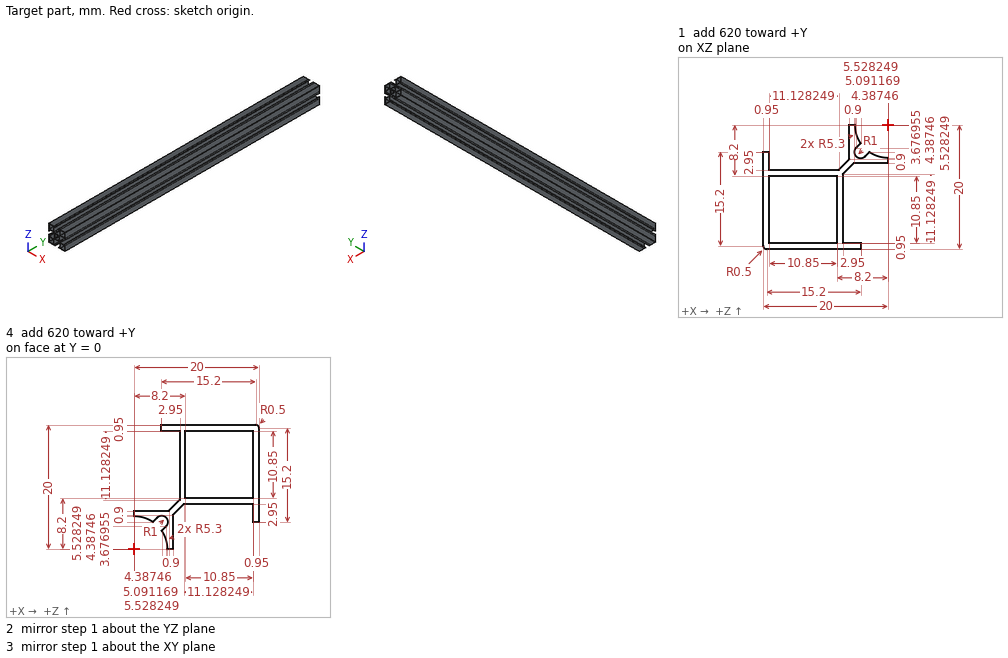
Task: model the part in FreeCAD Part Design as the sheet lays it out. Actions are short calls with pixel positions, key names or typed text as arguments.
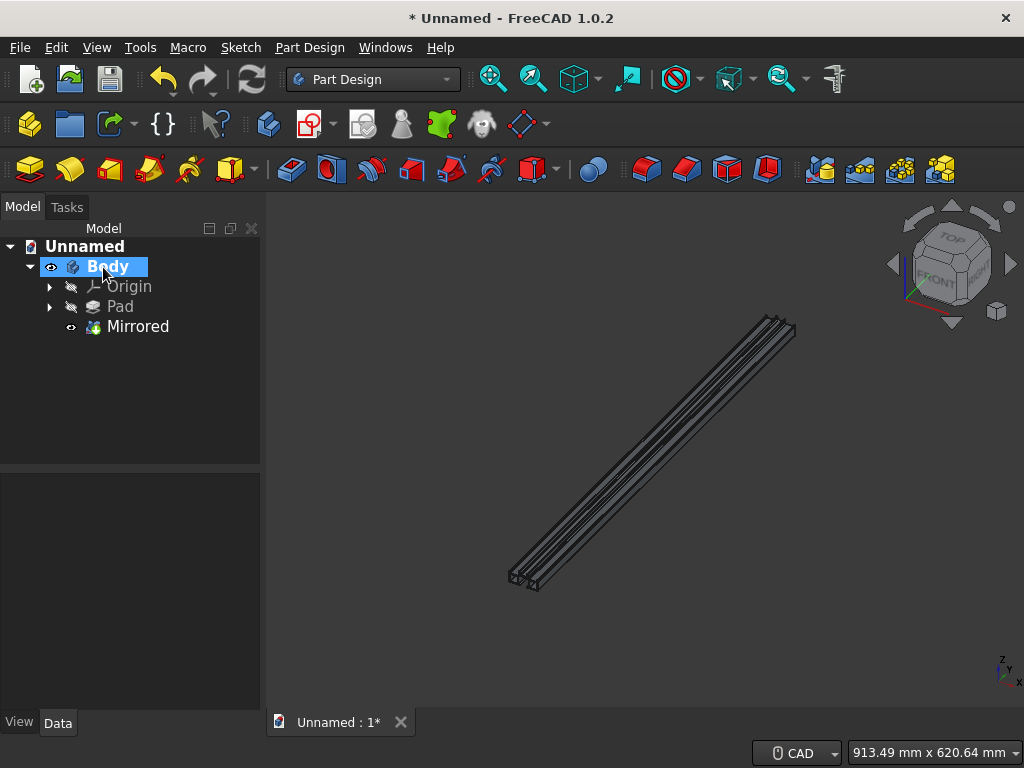
click(116, 307)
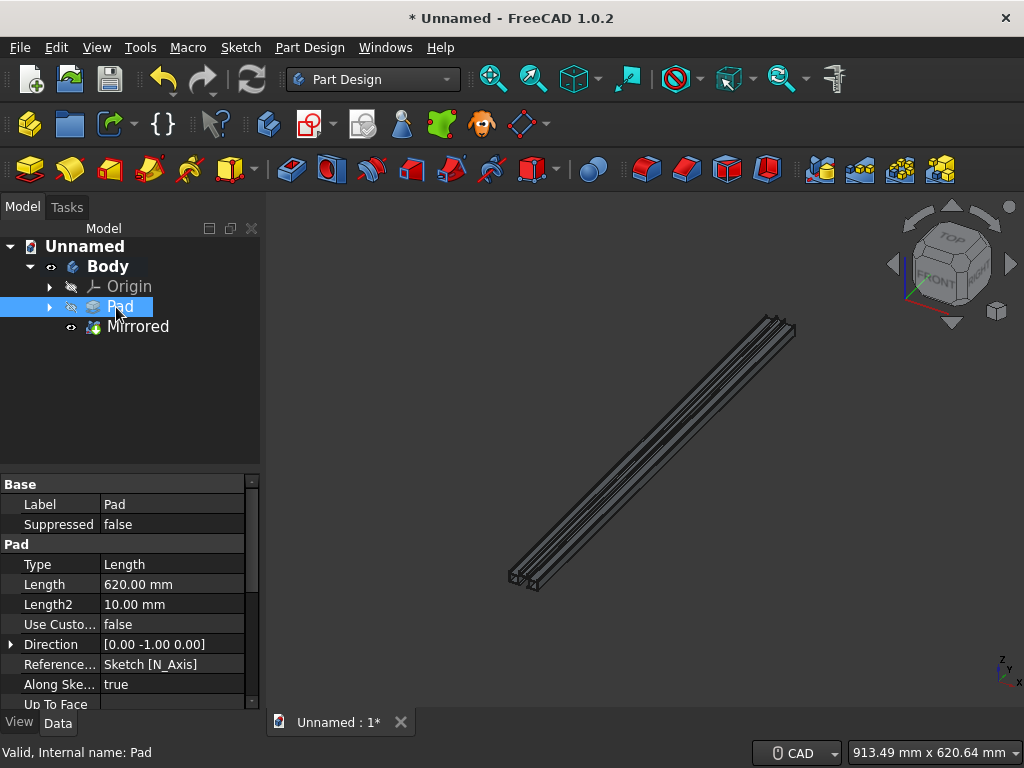
click(820, 170)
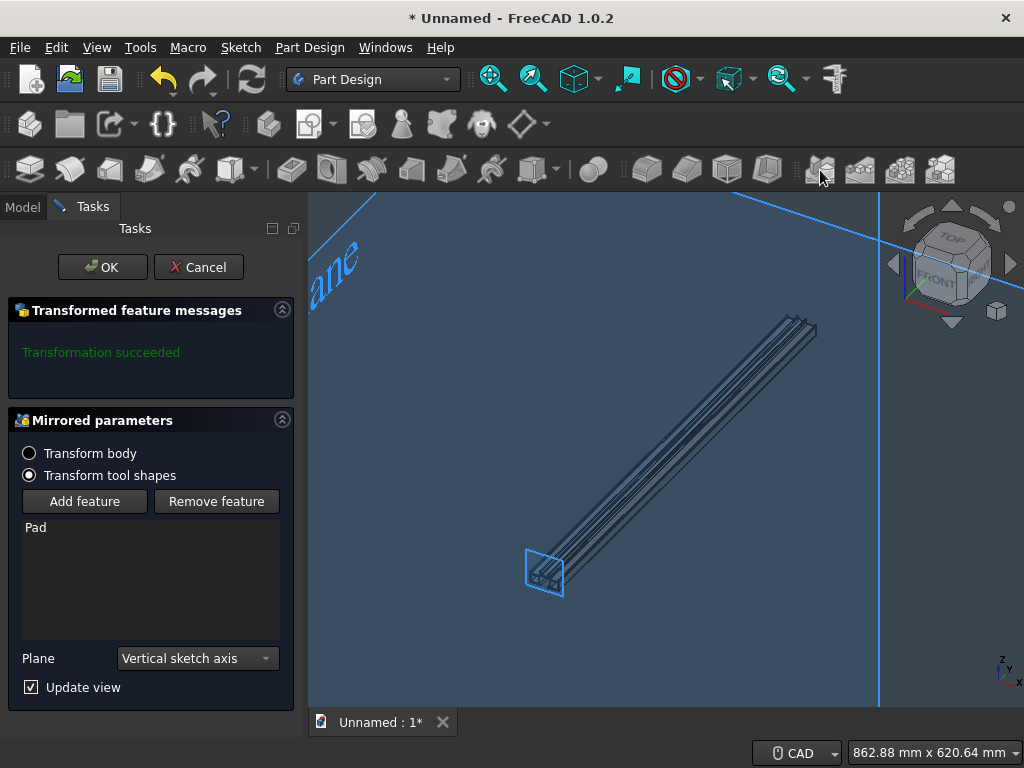
click(198, 658)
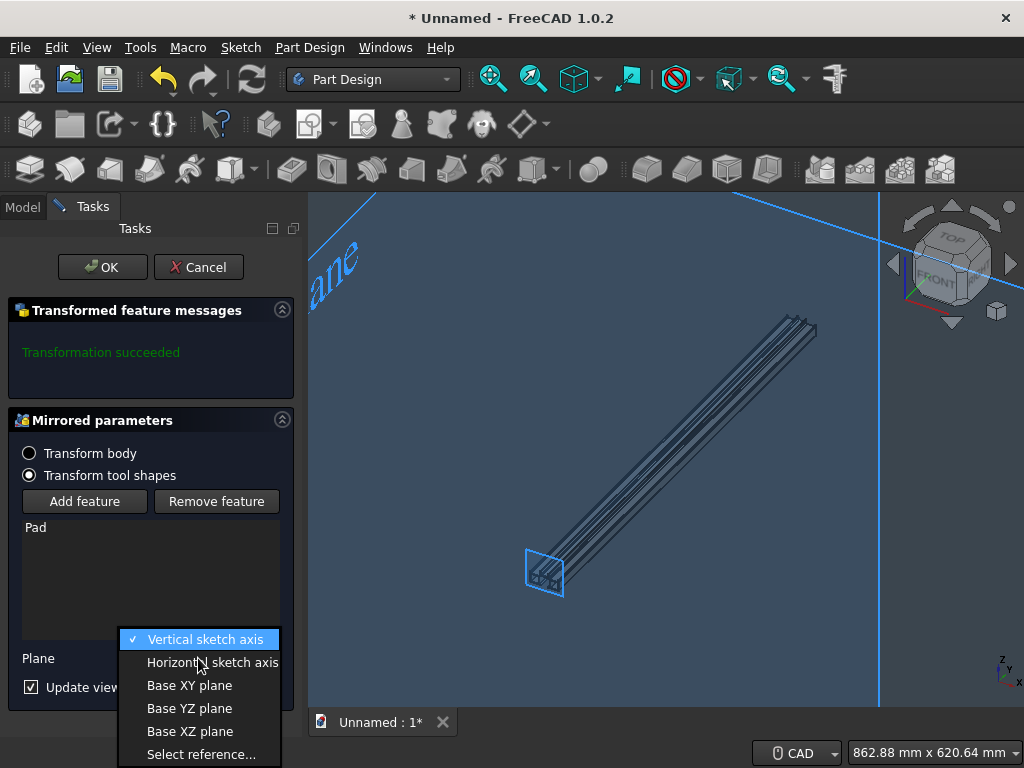
click(198, 686)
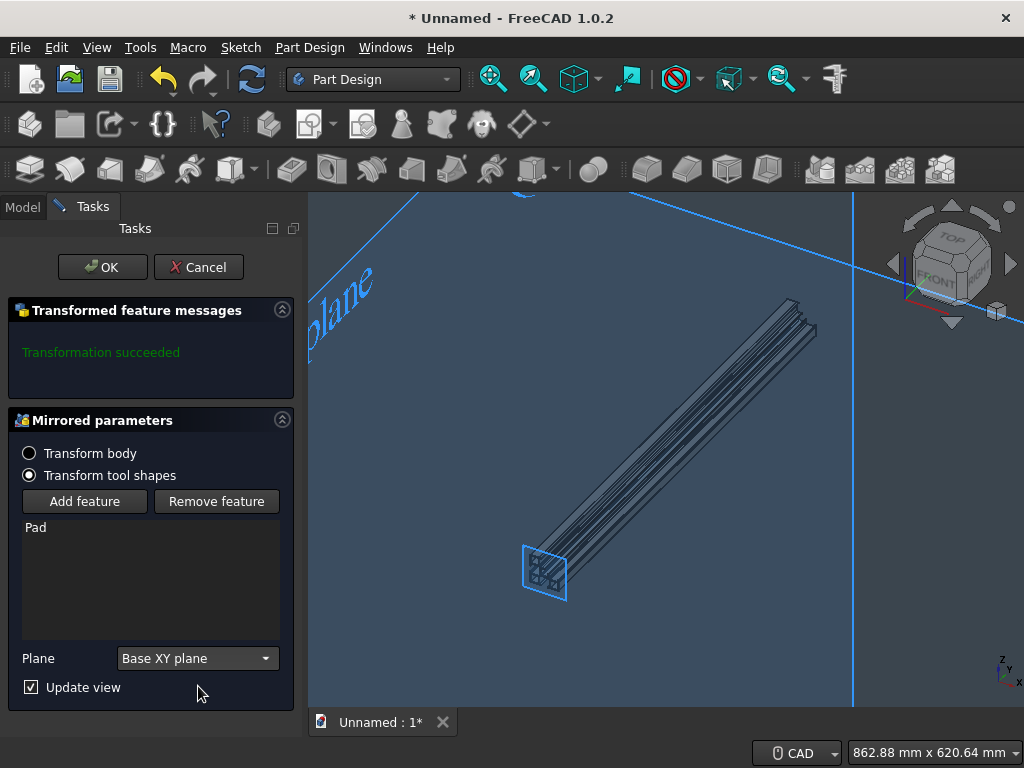
click(103, 267)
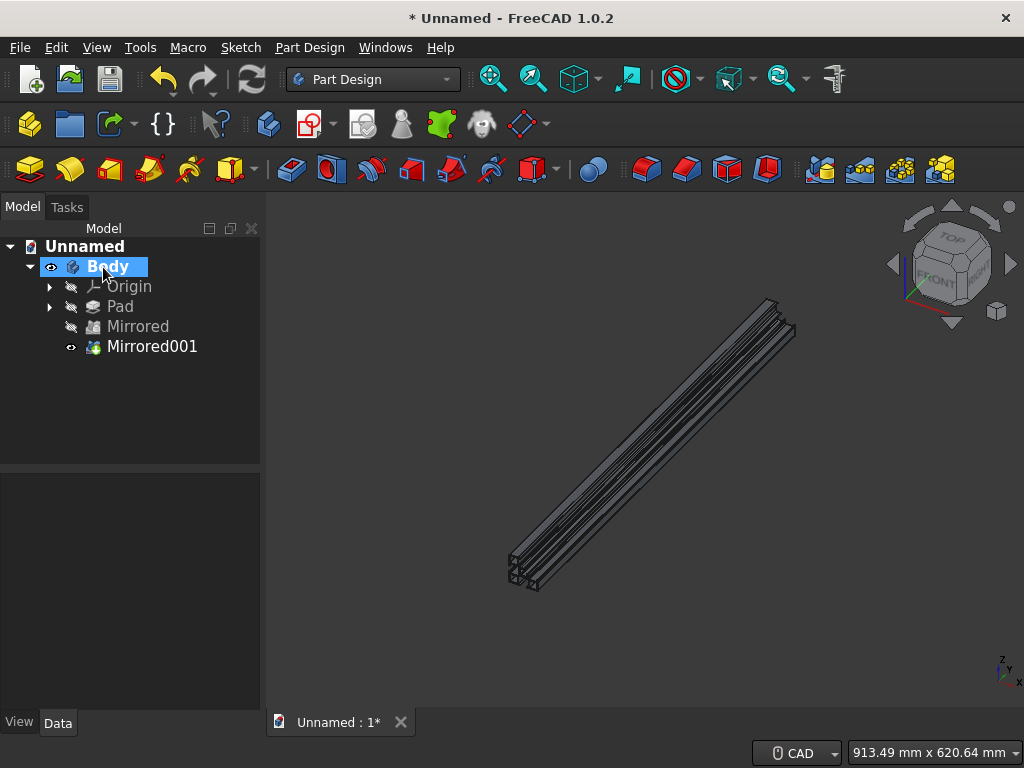
scroll(519, 574, up, 15)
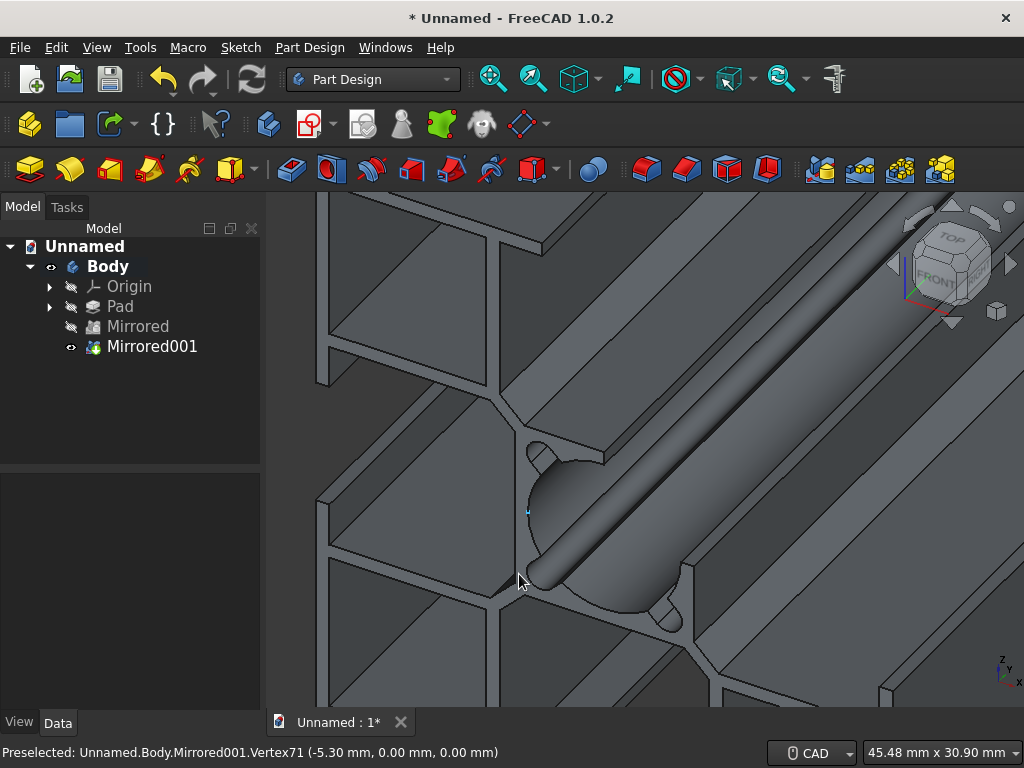
click(522, 587)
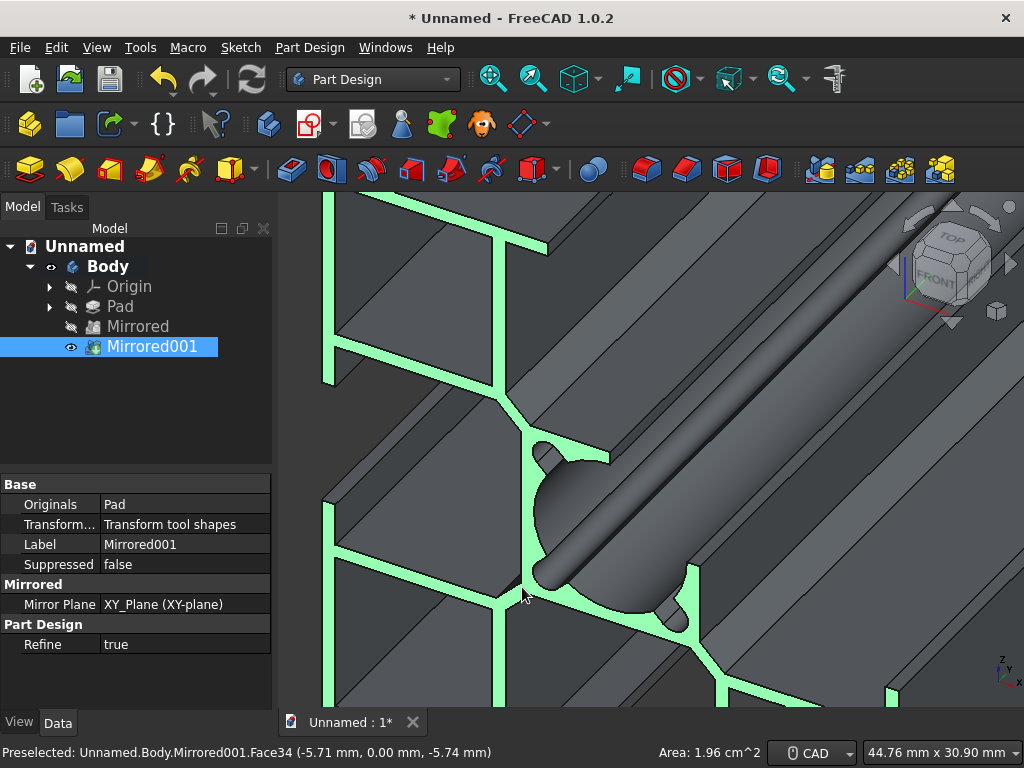
click(310, 124)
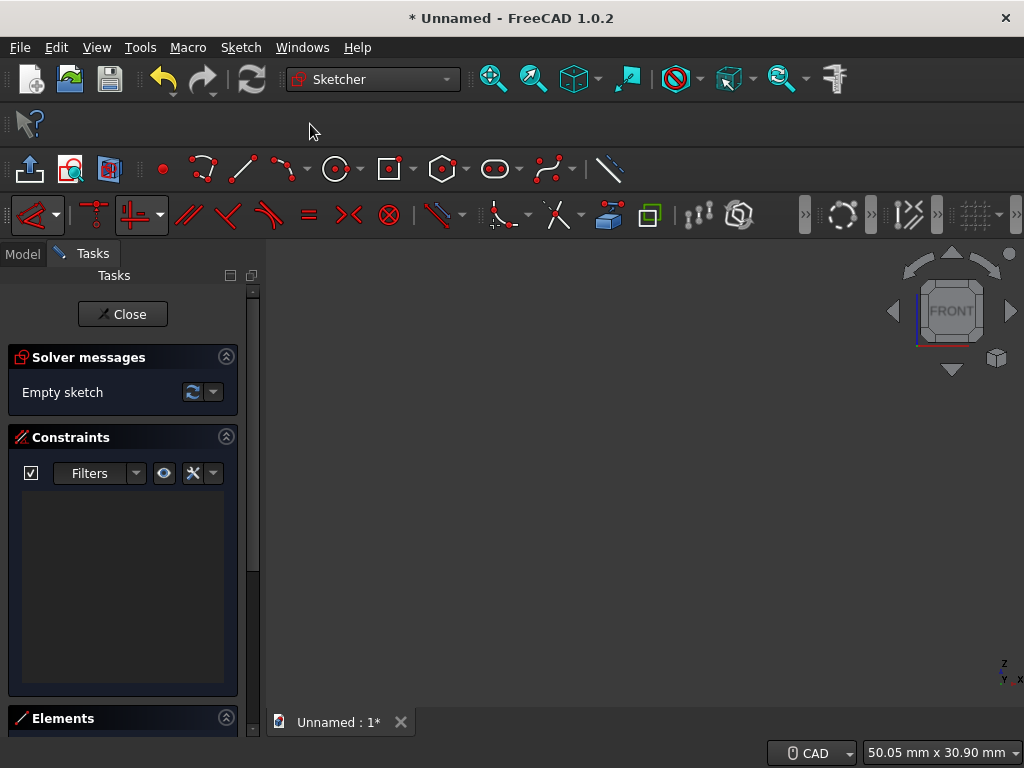
scroll(576, 473, down, 5)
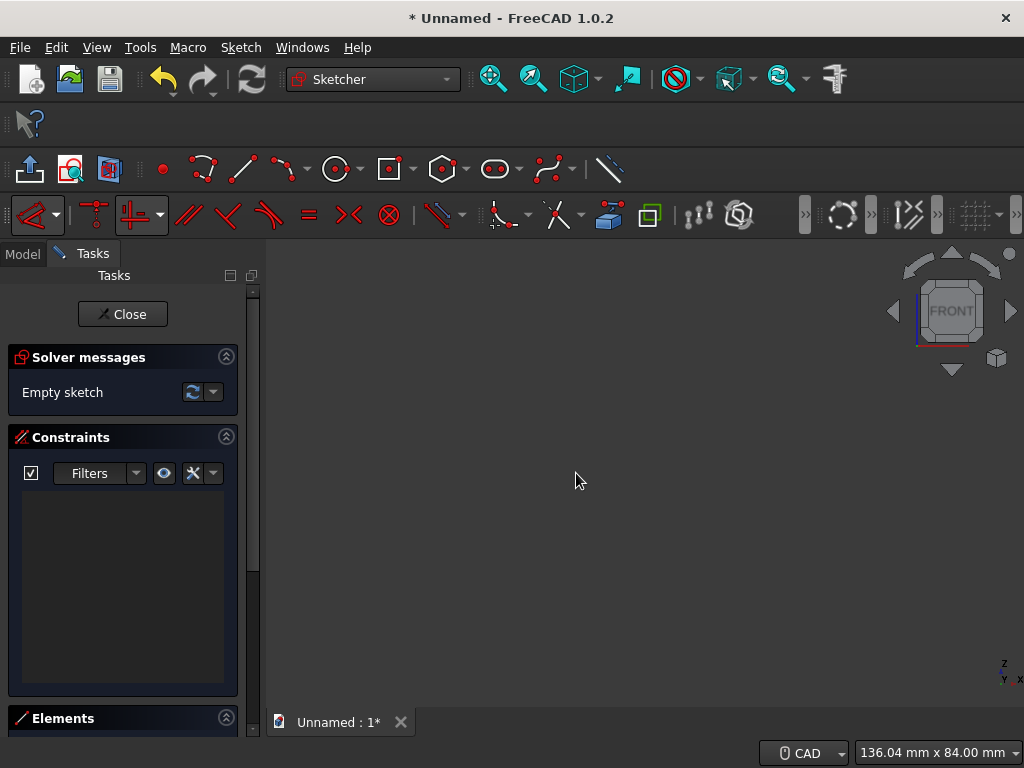
scroll(576, 473, down, 5)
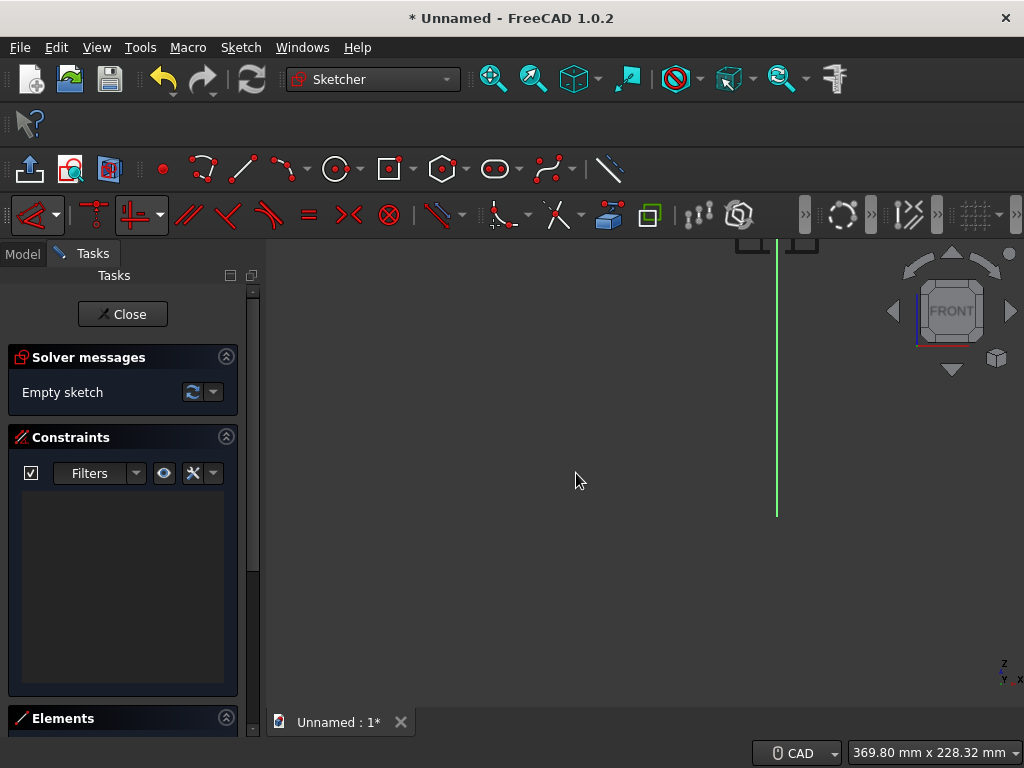
scroll(576, 473, down, 5)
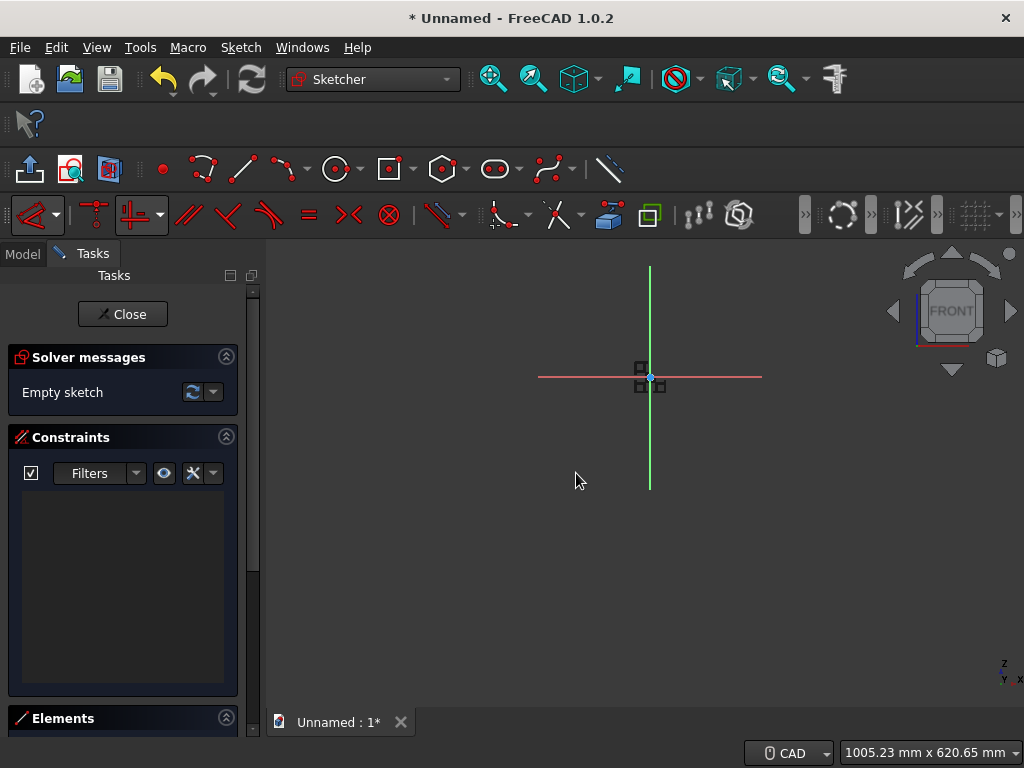
scroll(662, 364, up, 15)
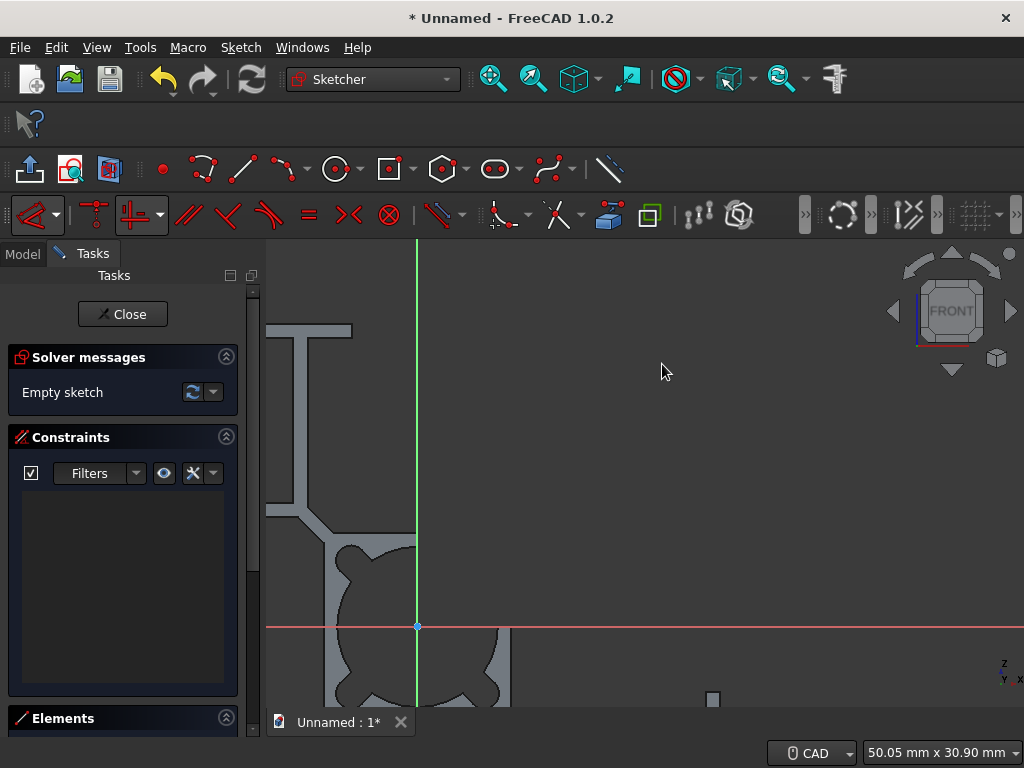
click(204, 170)